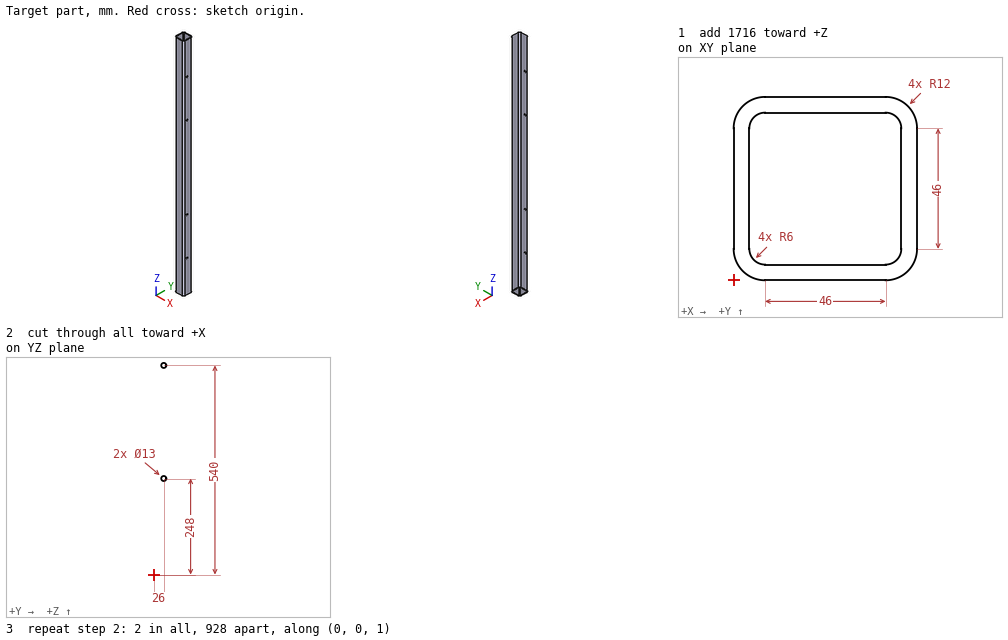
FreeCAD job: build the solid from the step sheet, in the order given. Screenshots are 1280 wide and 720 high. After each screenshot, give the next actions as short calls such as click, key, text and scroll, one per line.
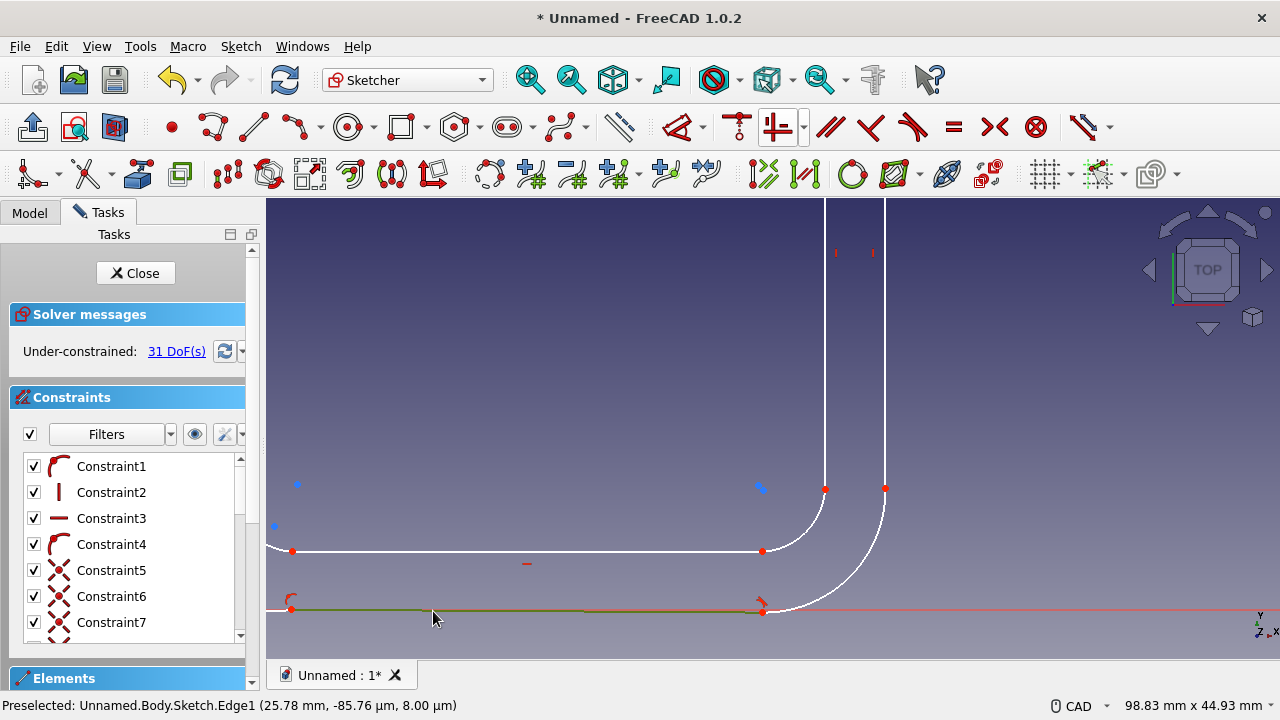
scroll(807, 532, down, 5)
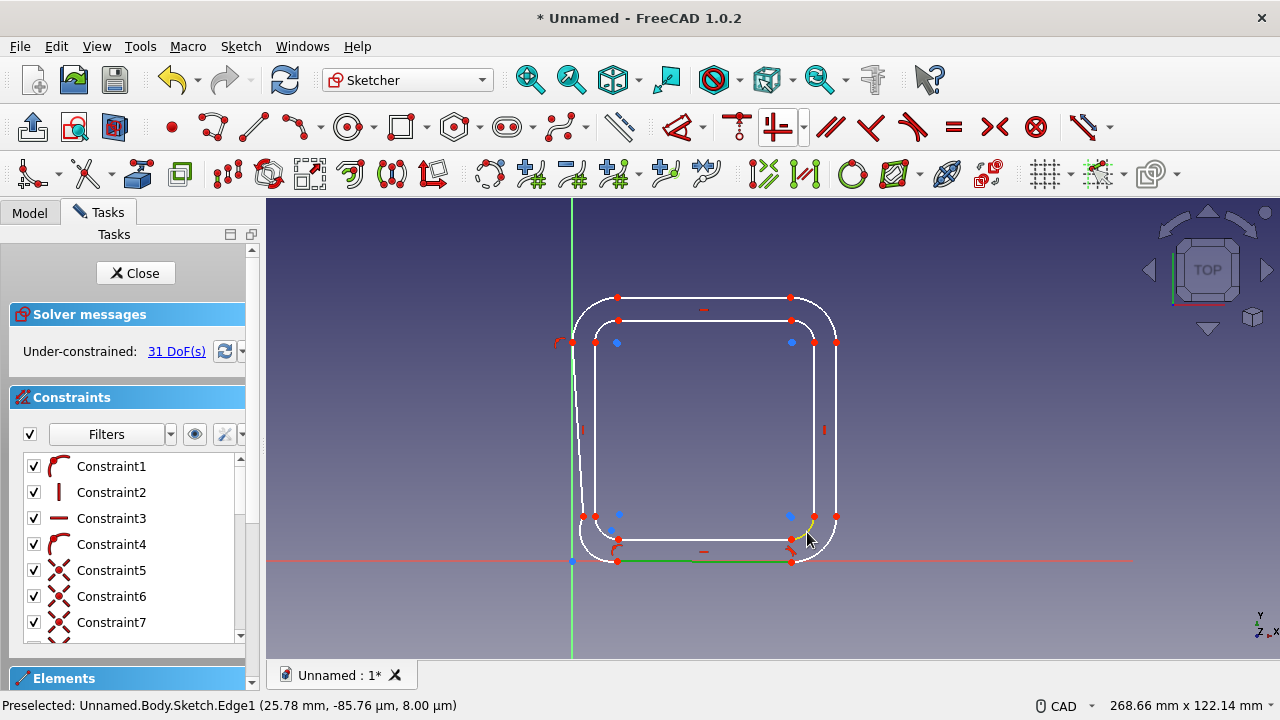
scroll(581, 537, up, 3)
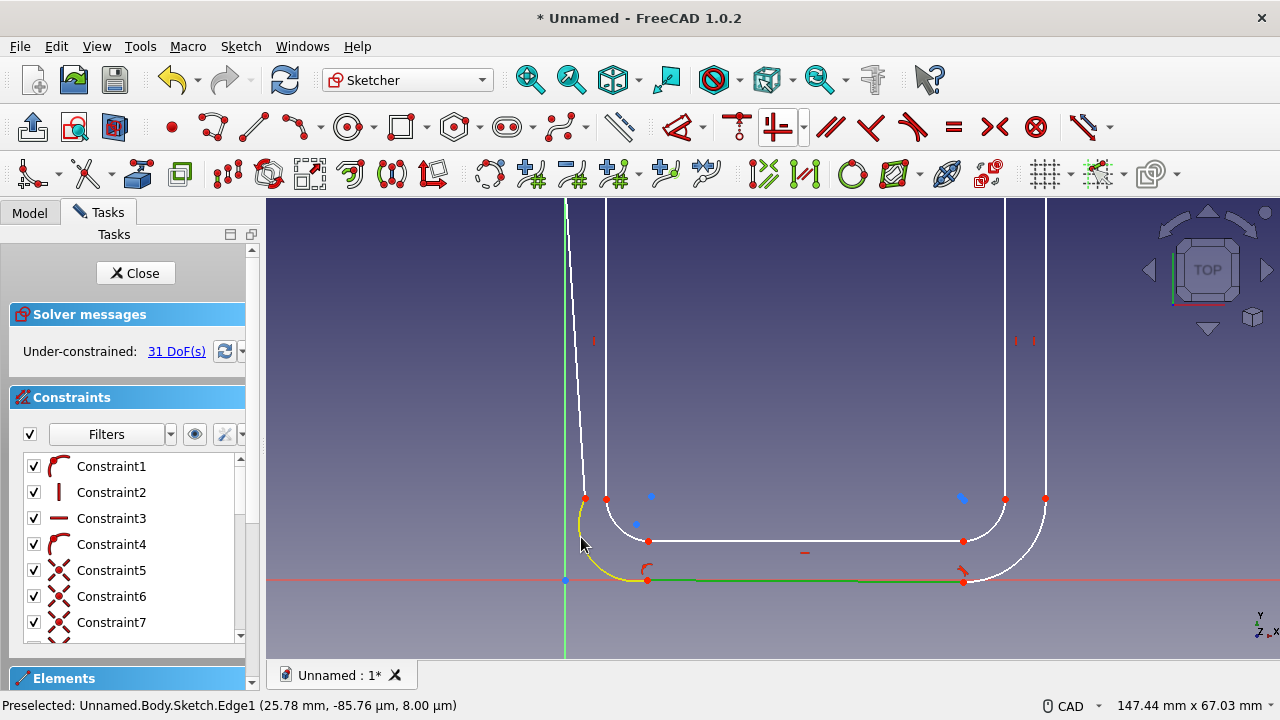
click(580, 536)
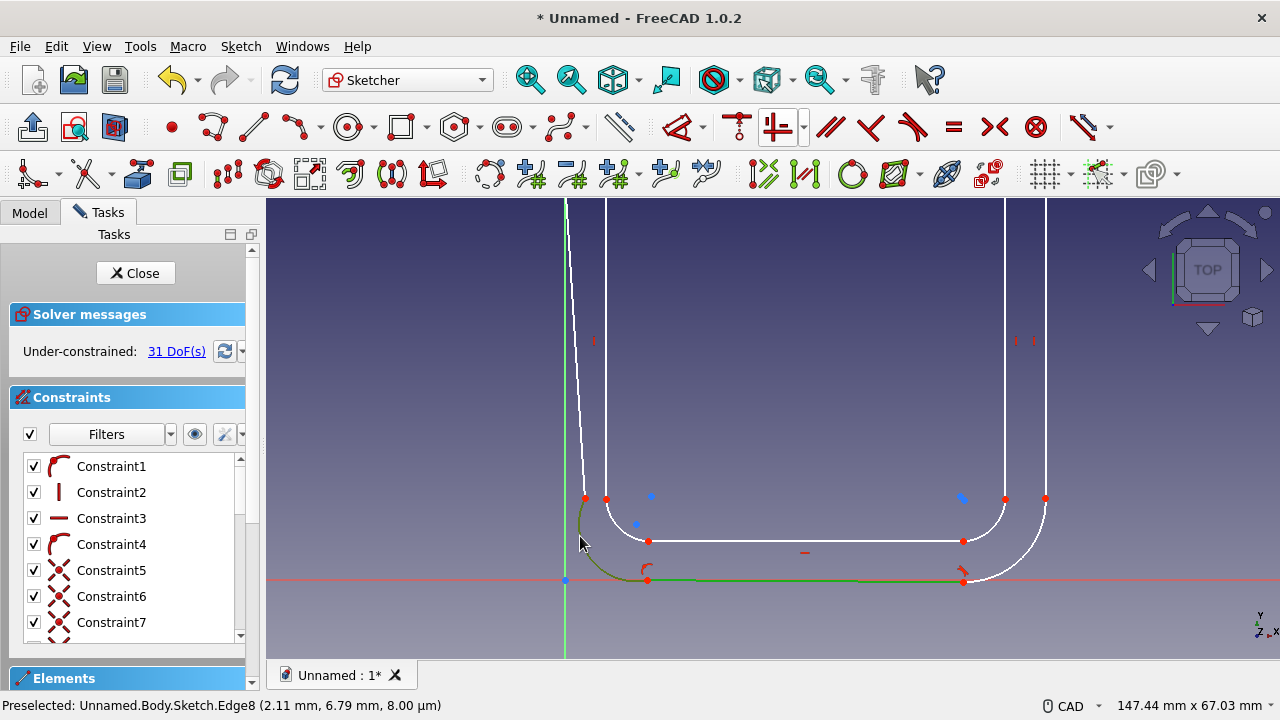
click(913, 128)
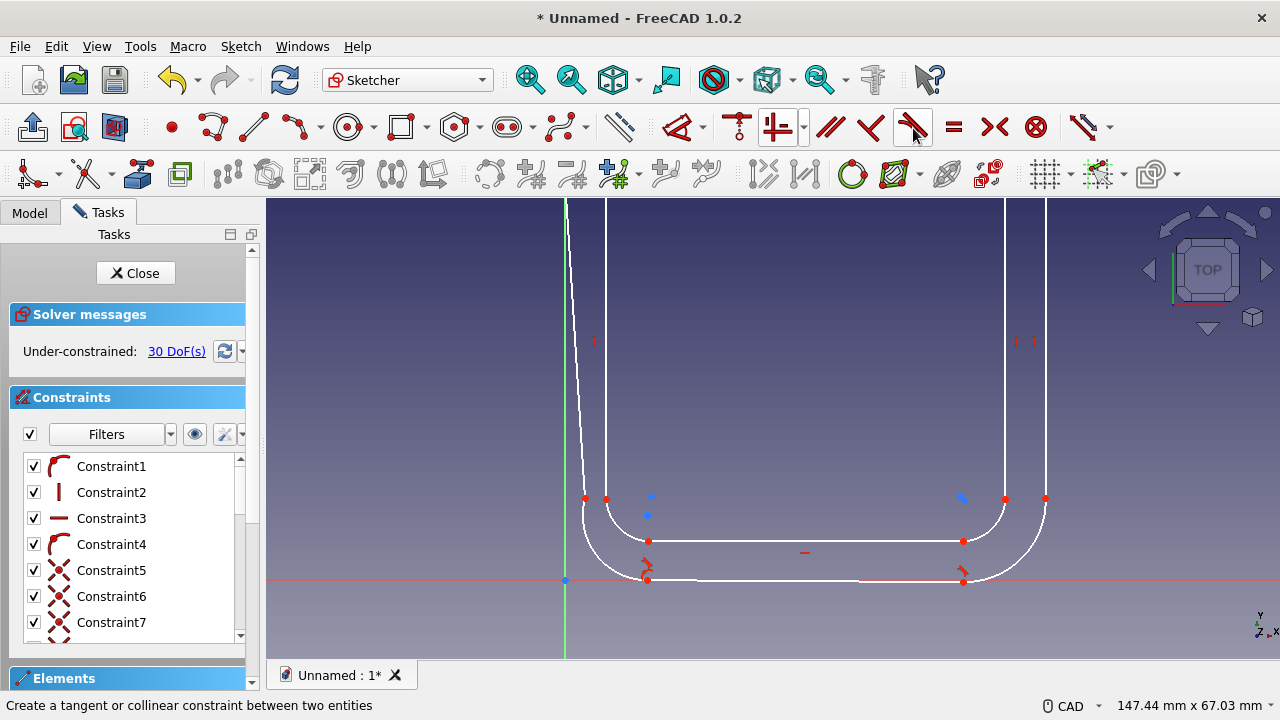
click(1046, 404)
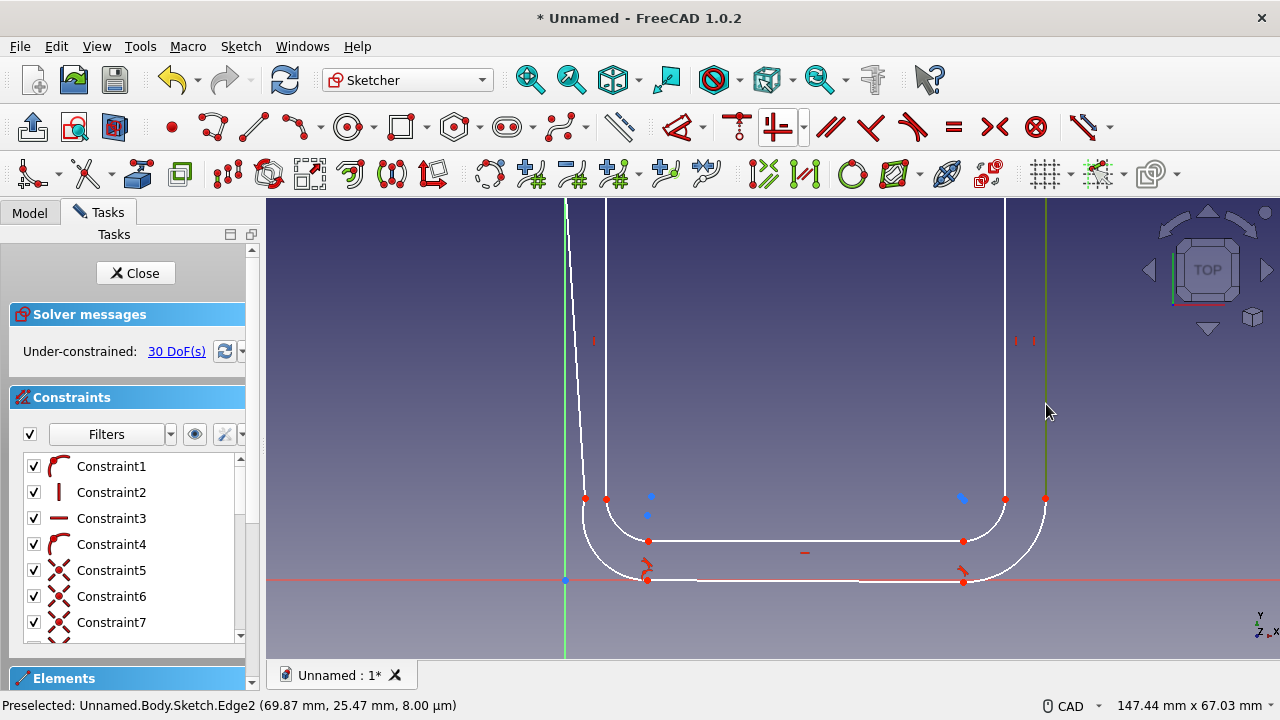
click(1037, 537)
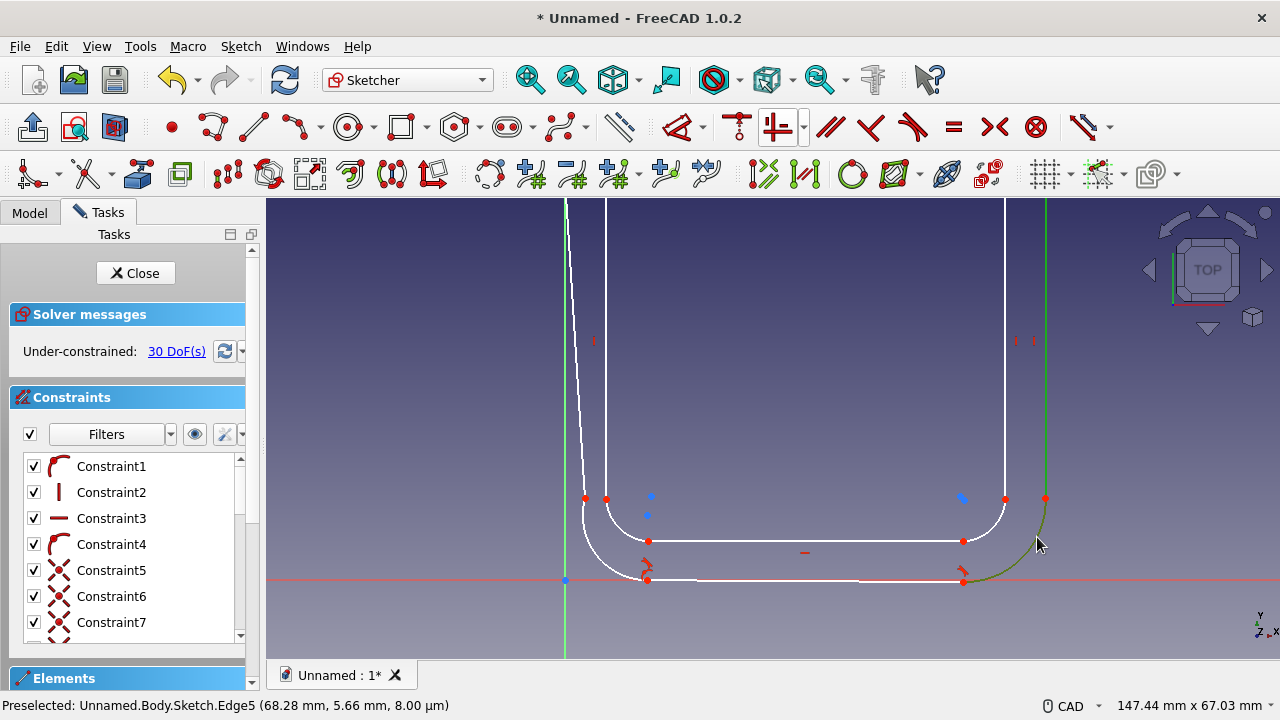
click(913, 128)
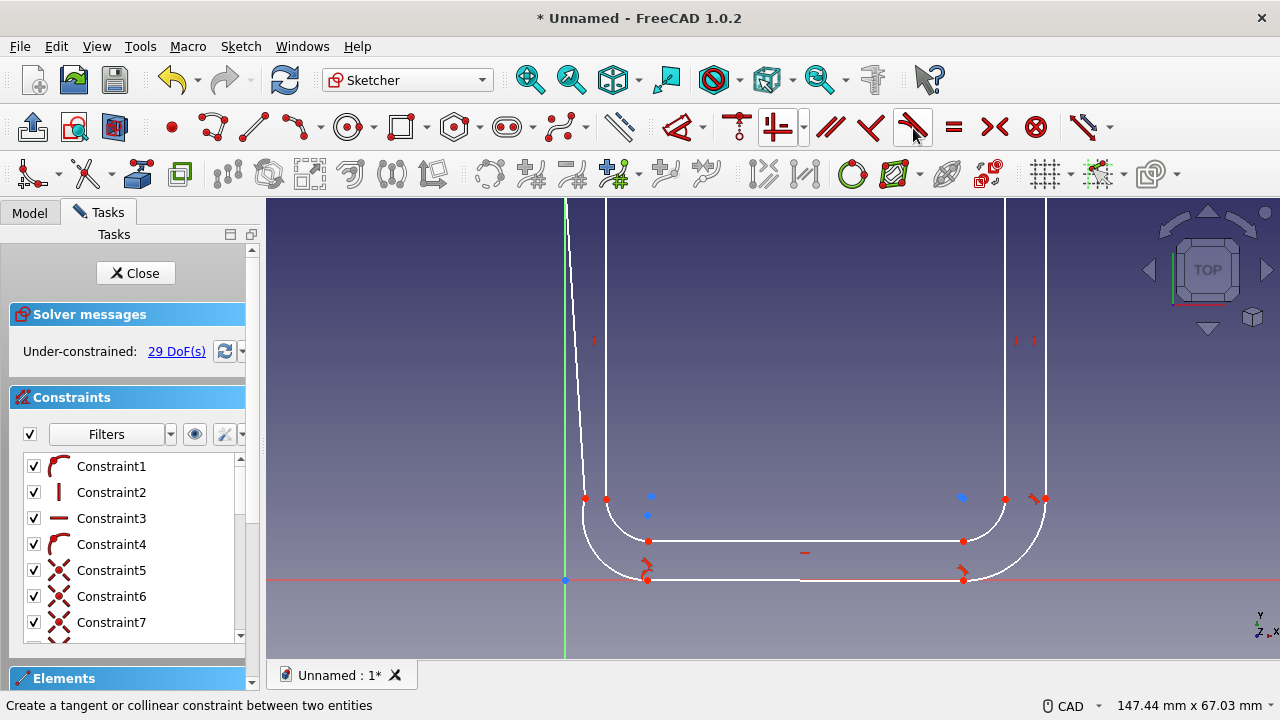
click(1046, 404)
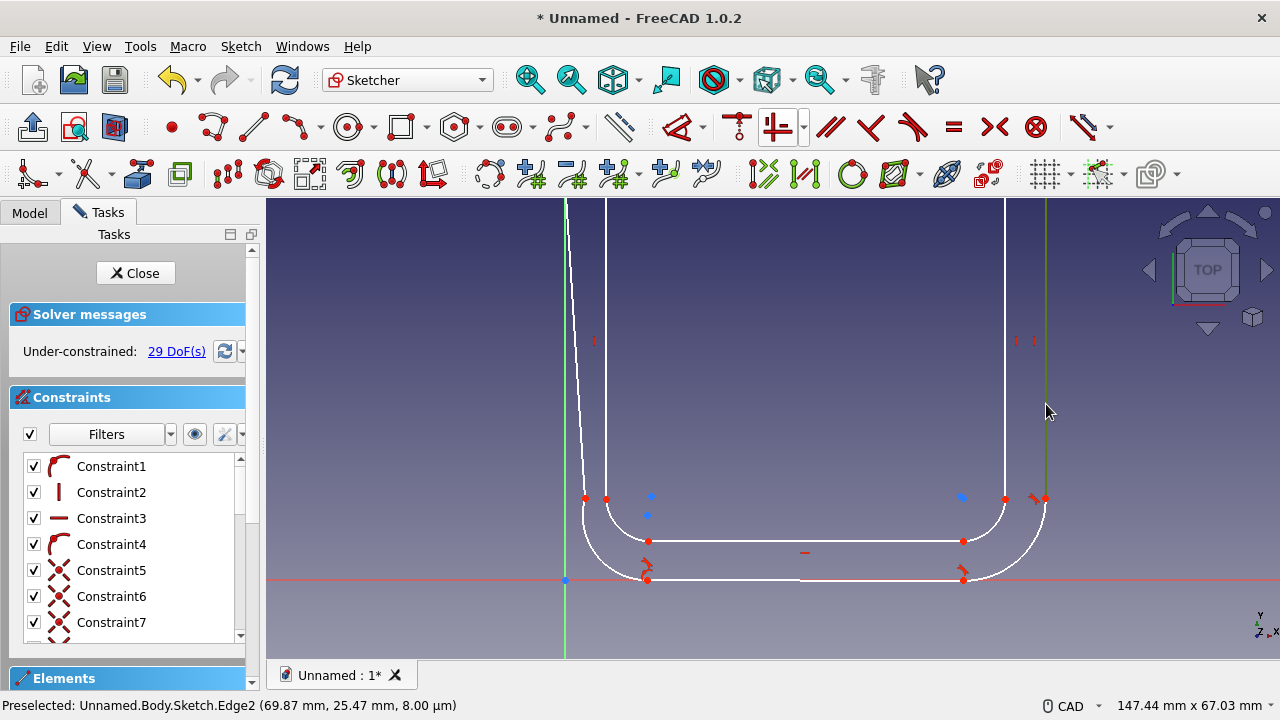
scroll(581, 537, down, 3)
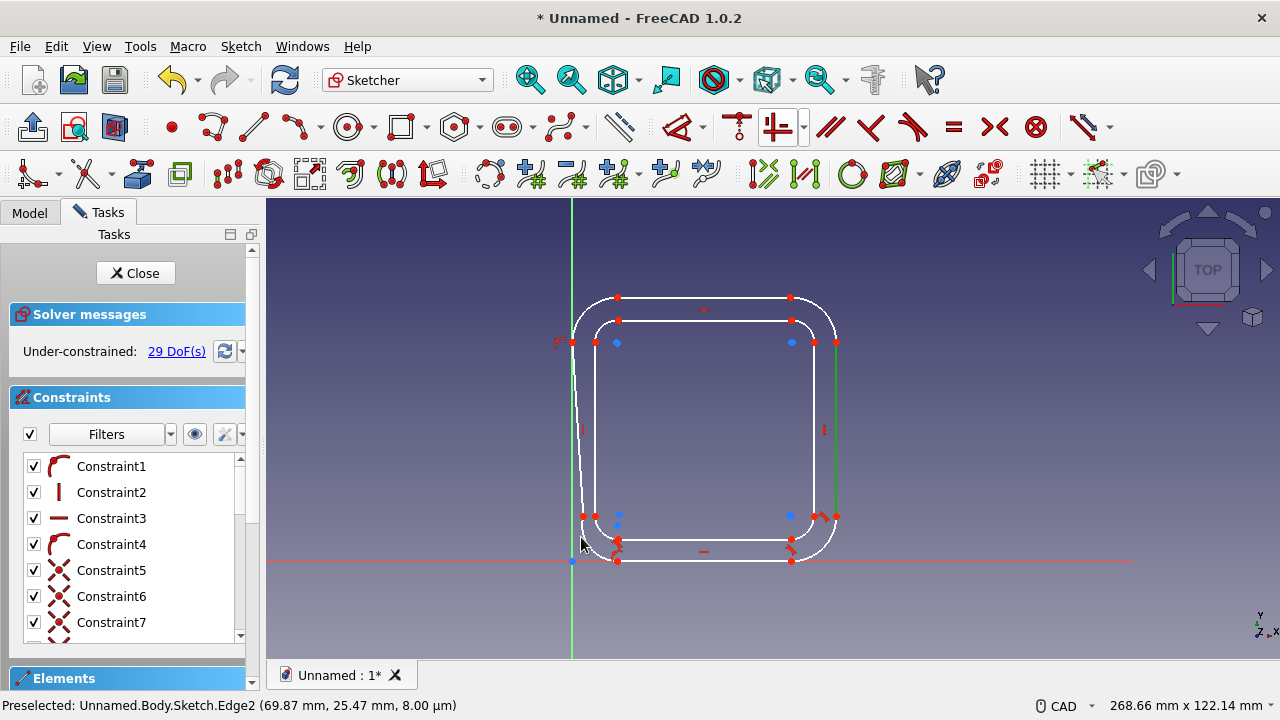
click(831, 322)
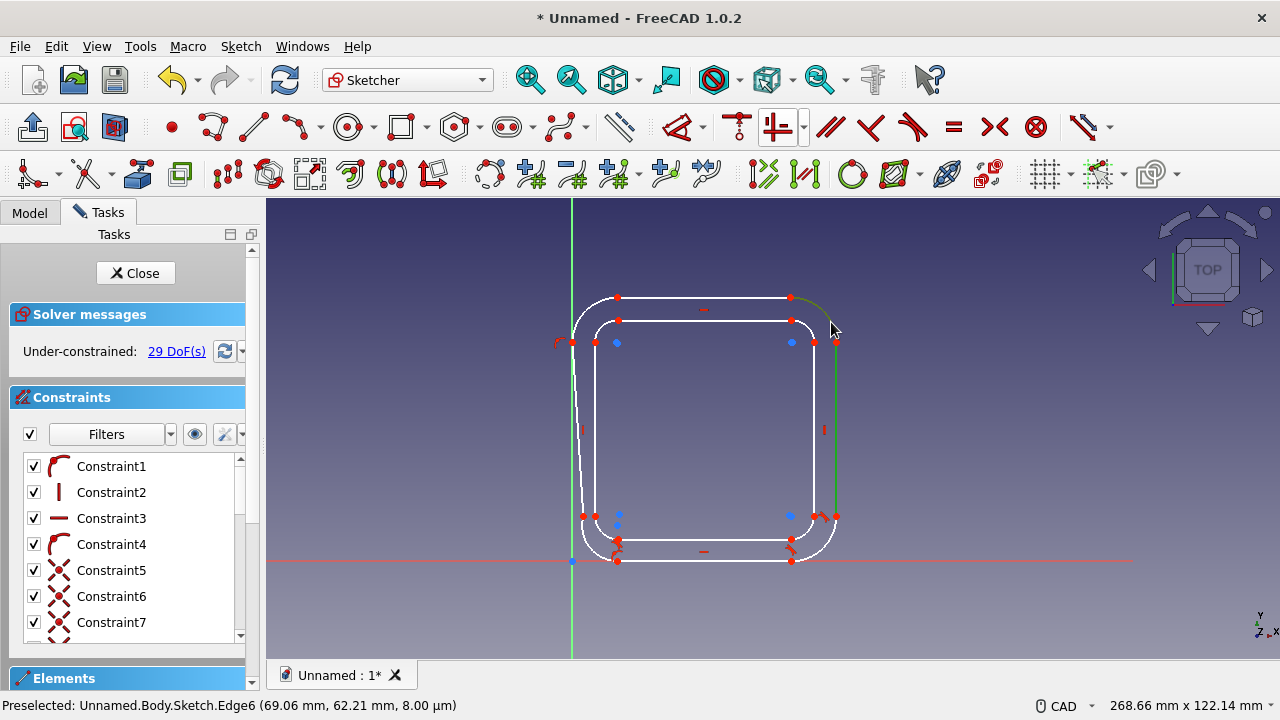
click(913, 128)